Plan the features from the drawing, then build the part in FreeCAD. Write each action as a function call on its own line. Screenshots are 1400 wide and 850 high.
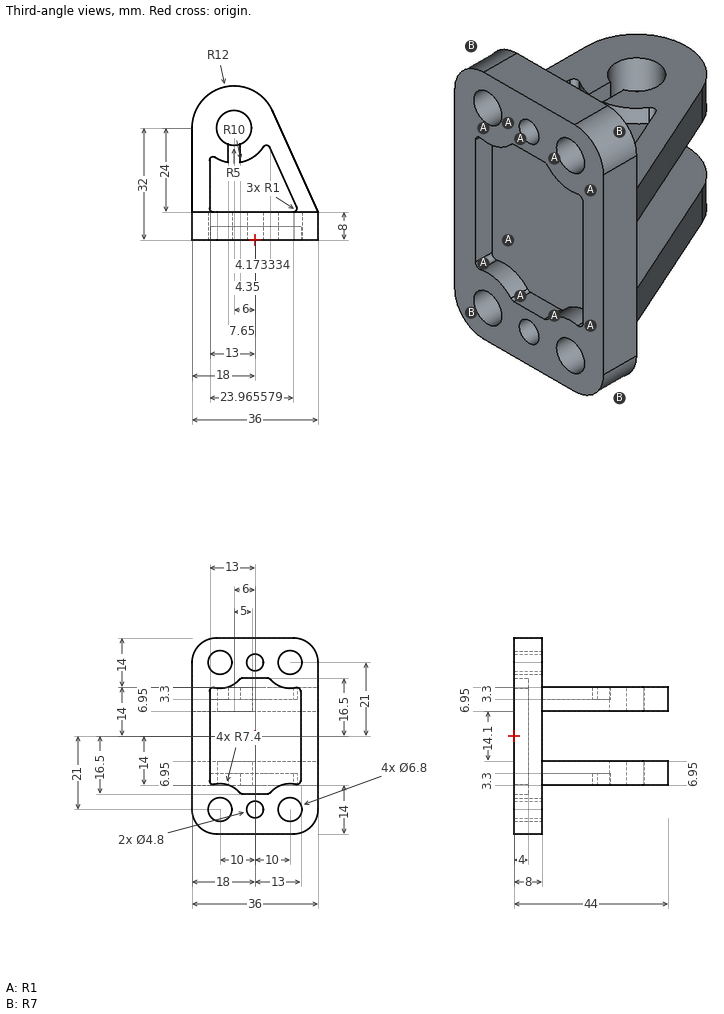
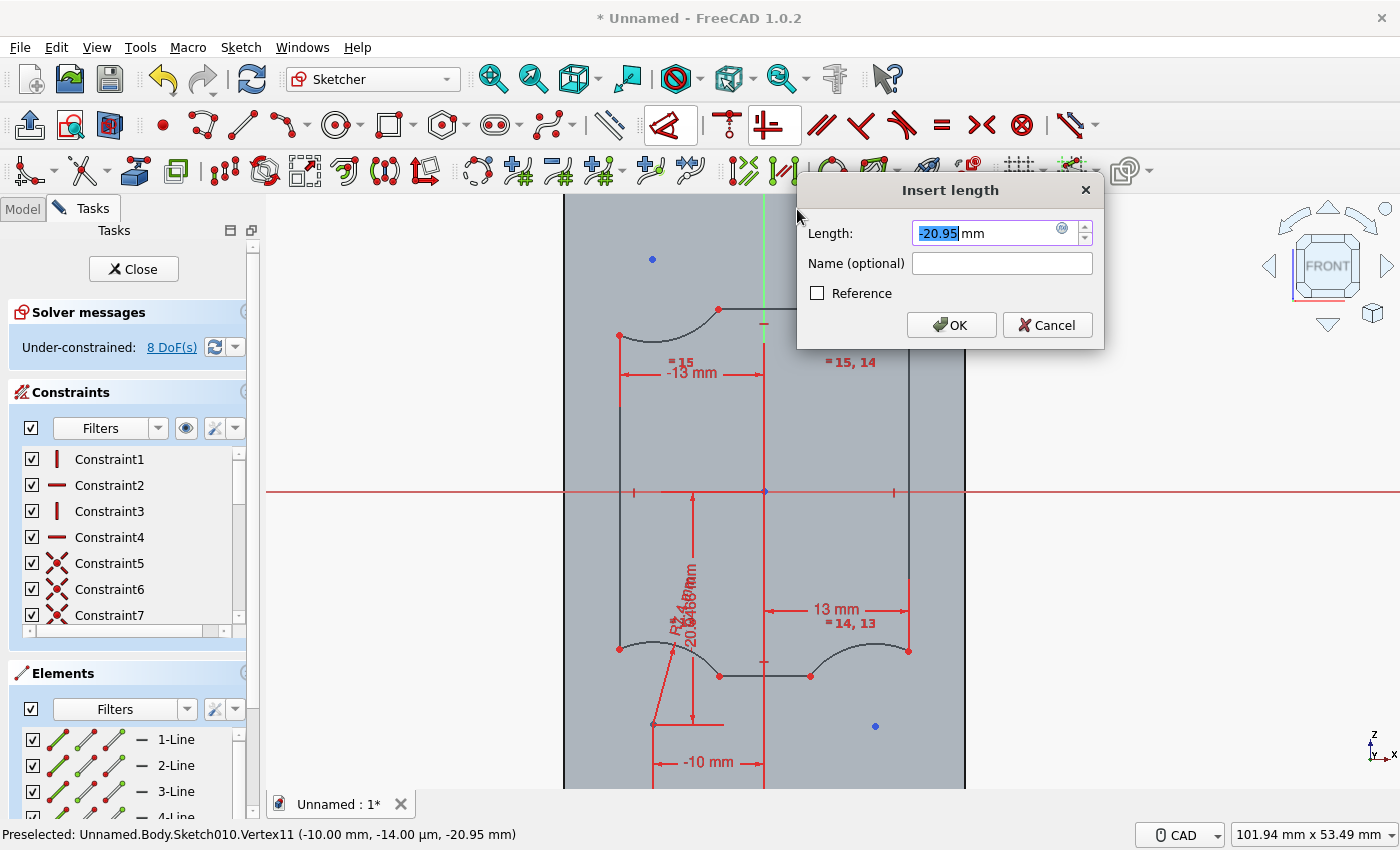
text(-21)
key(Return)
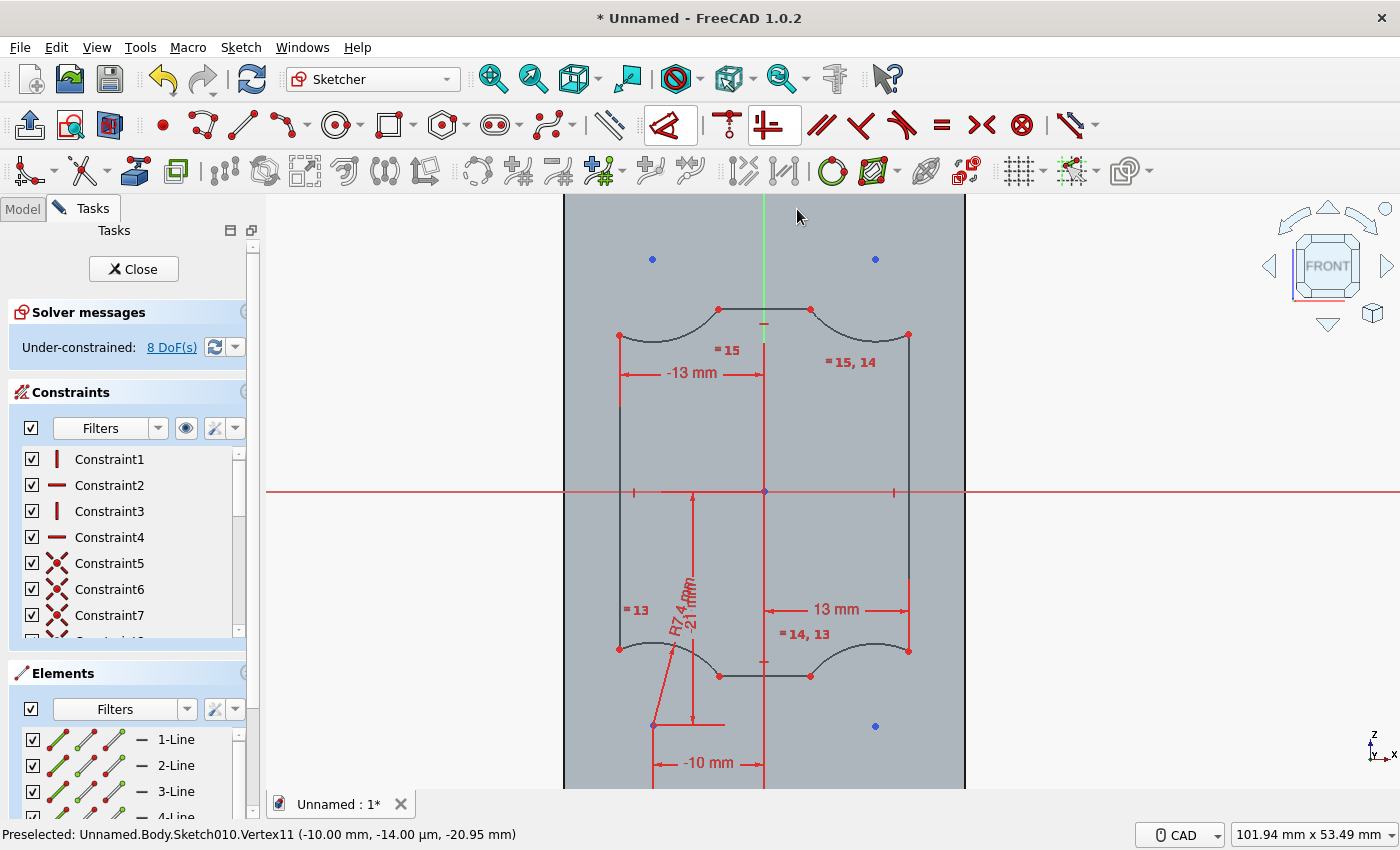
click(875, 726)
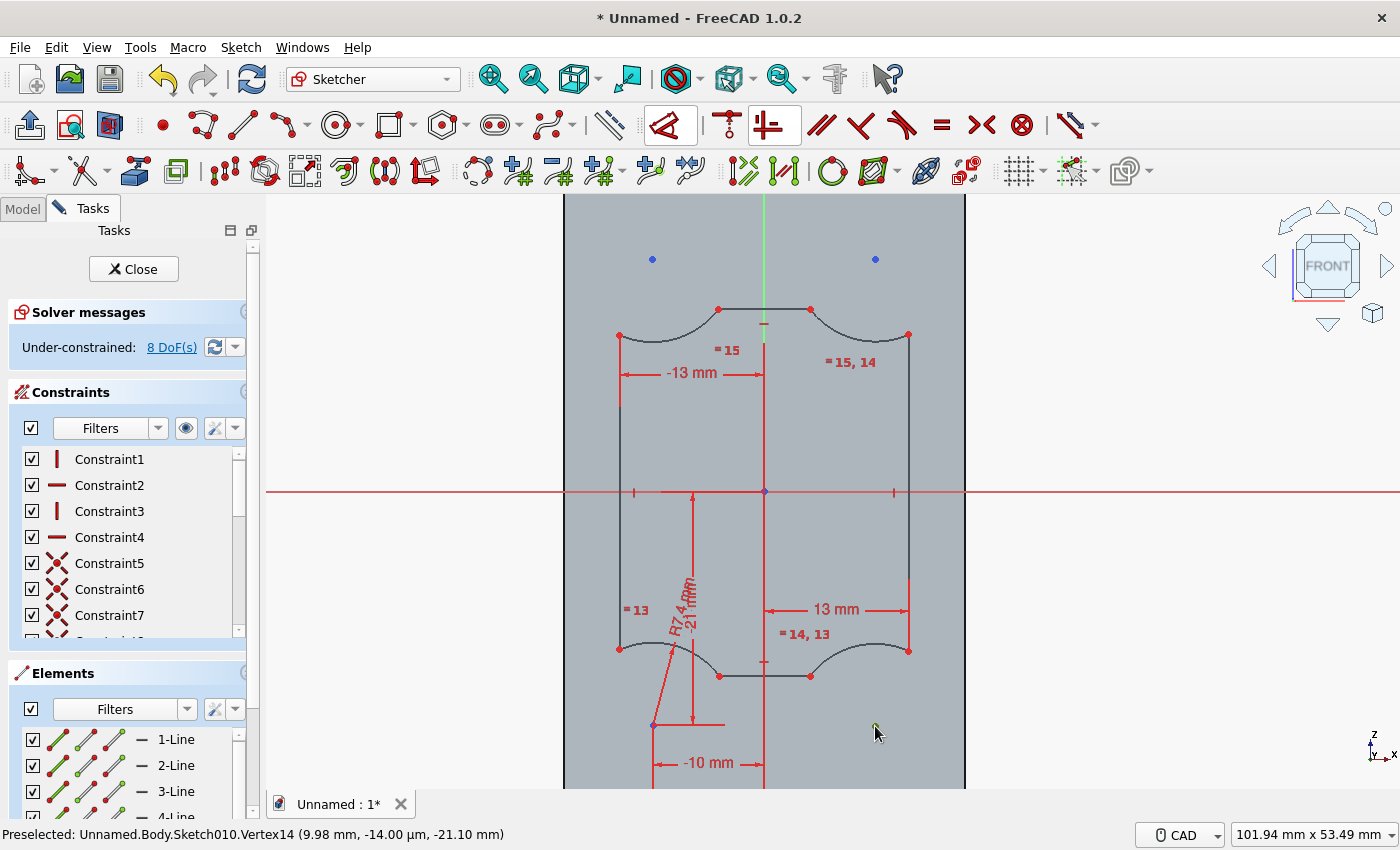
key(l)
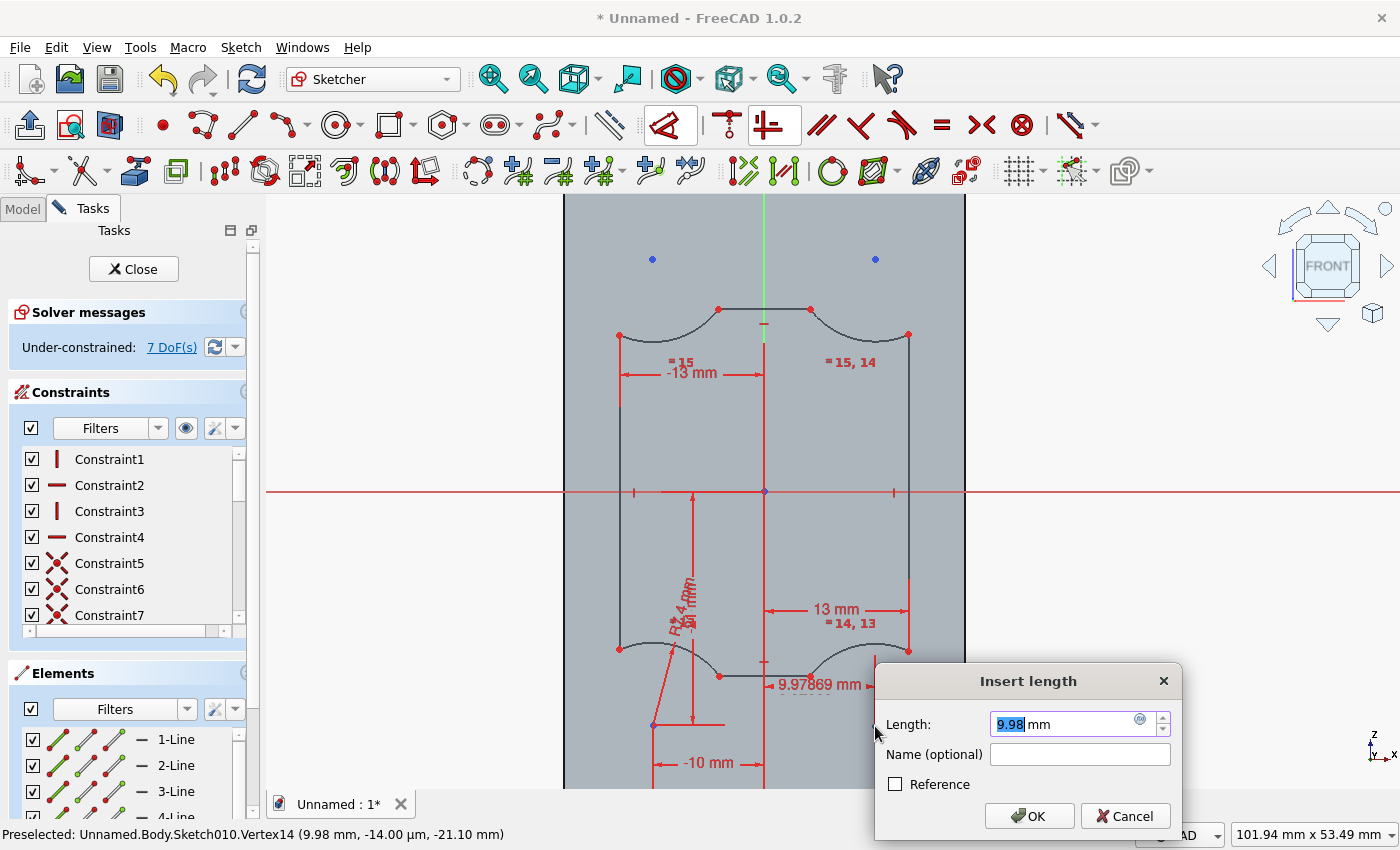
text(10)
key(Return)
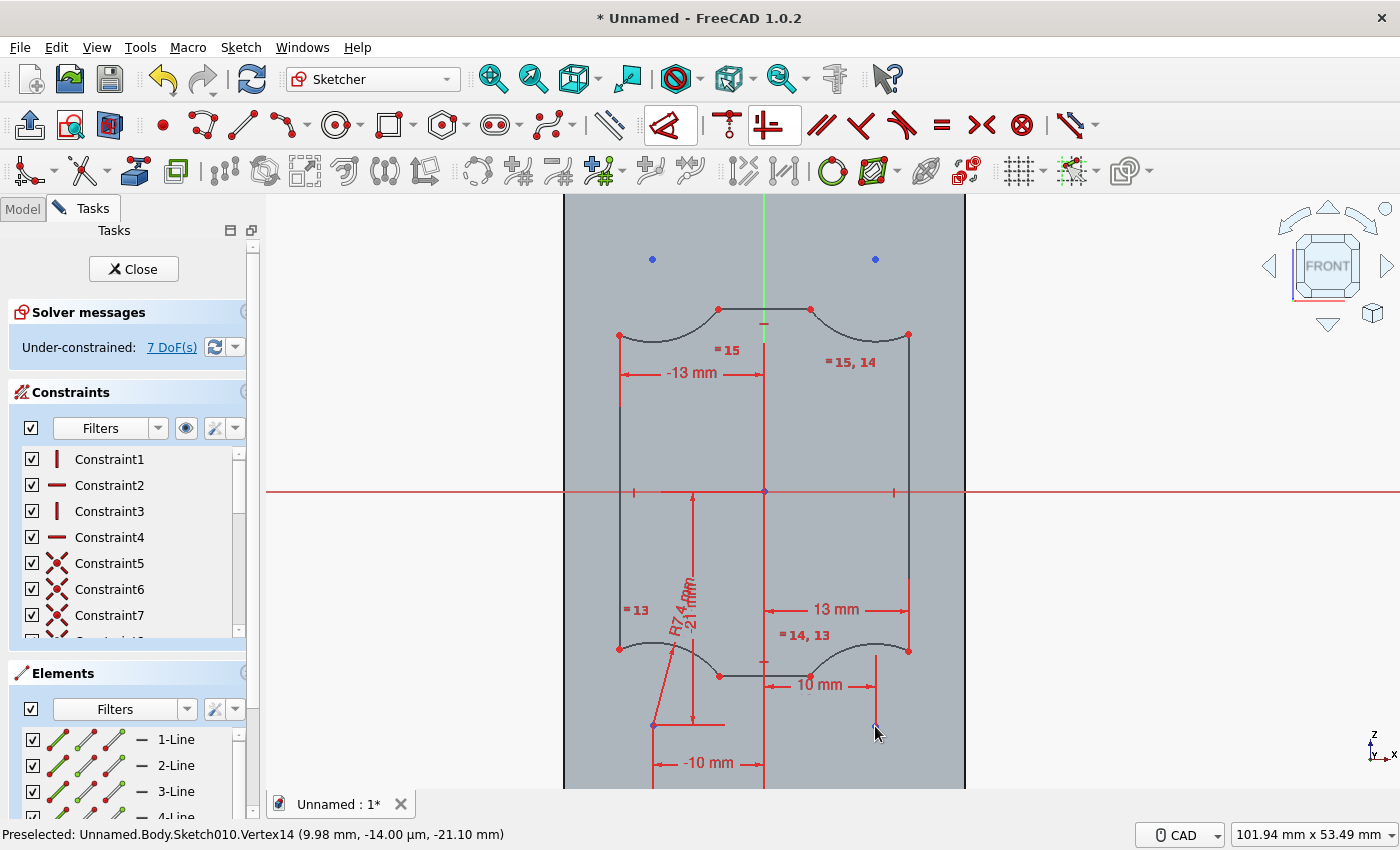
click(876, 726)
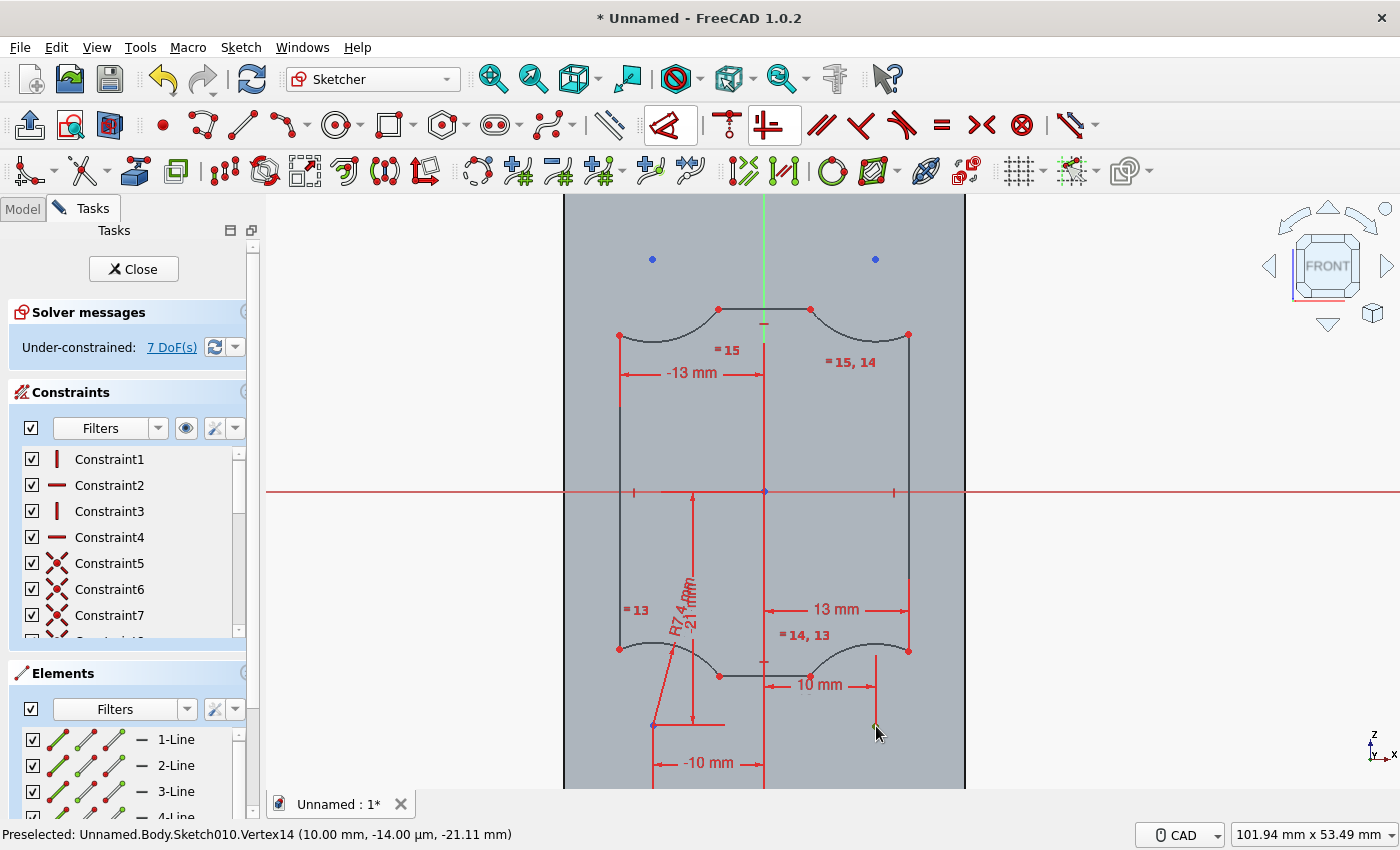
key(i)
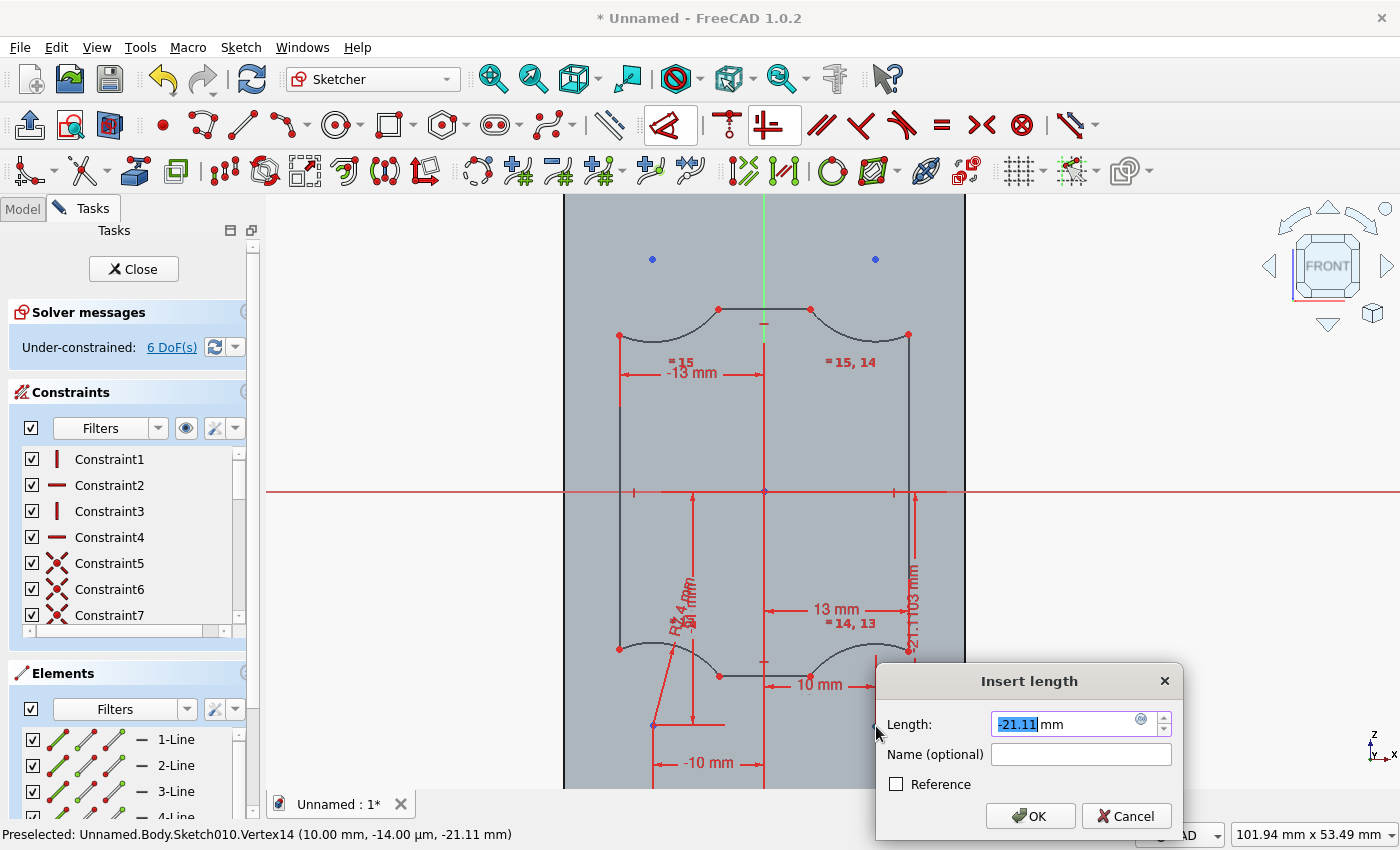
text(-21)
key(Return)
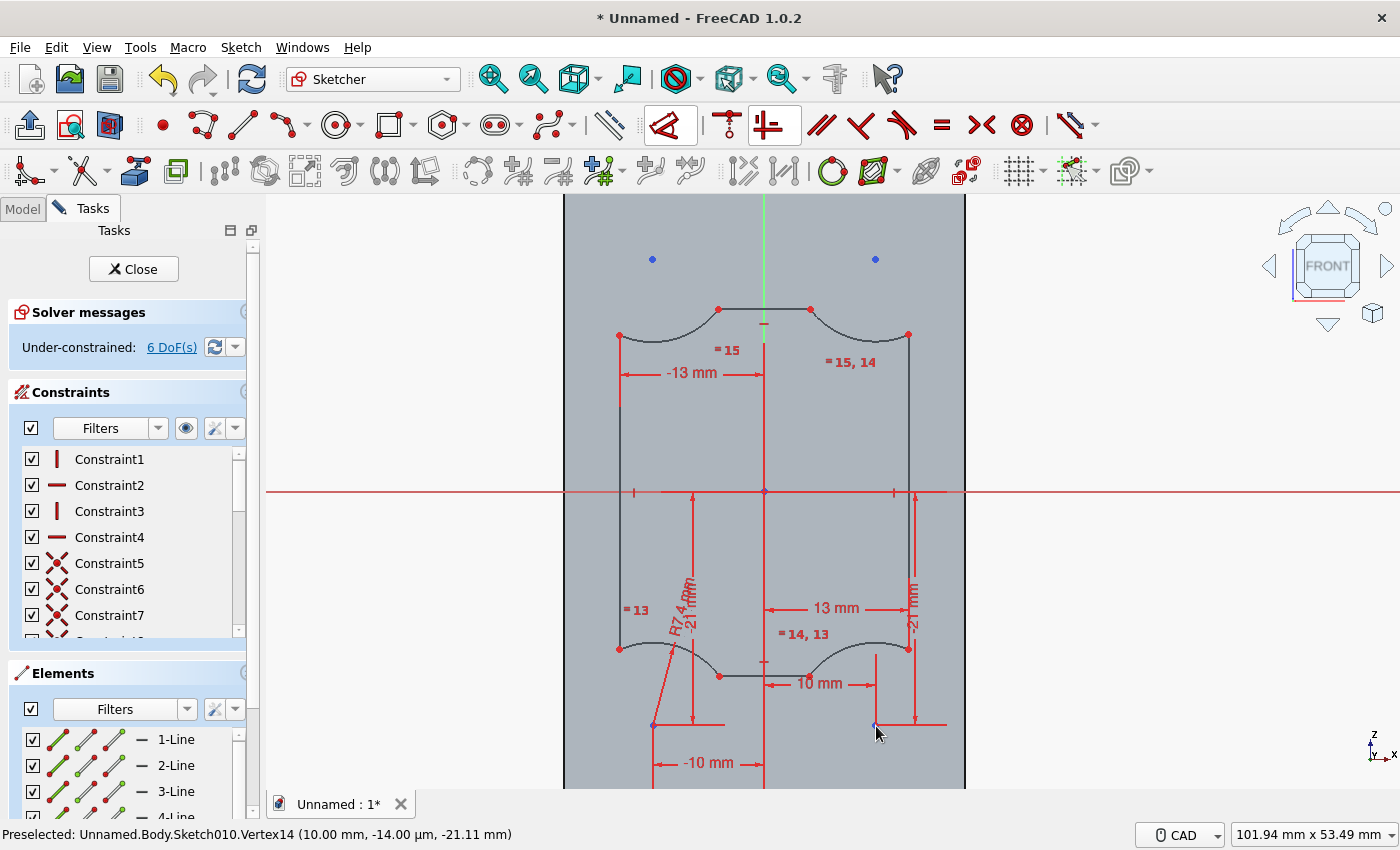
click(876, 259)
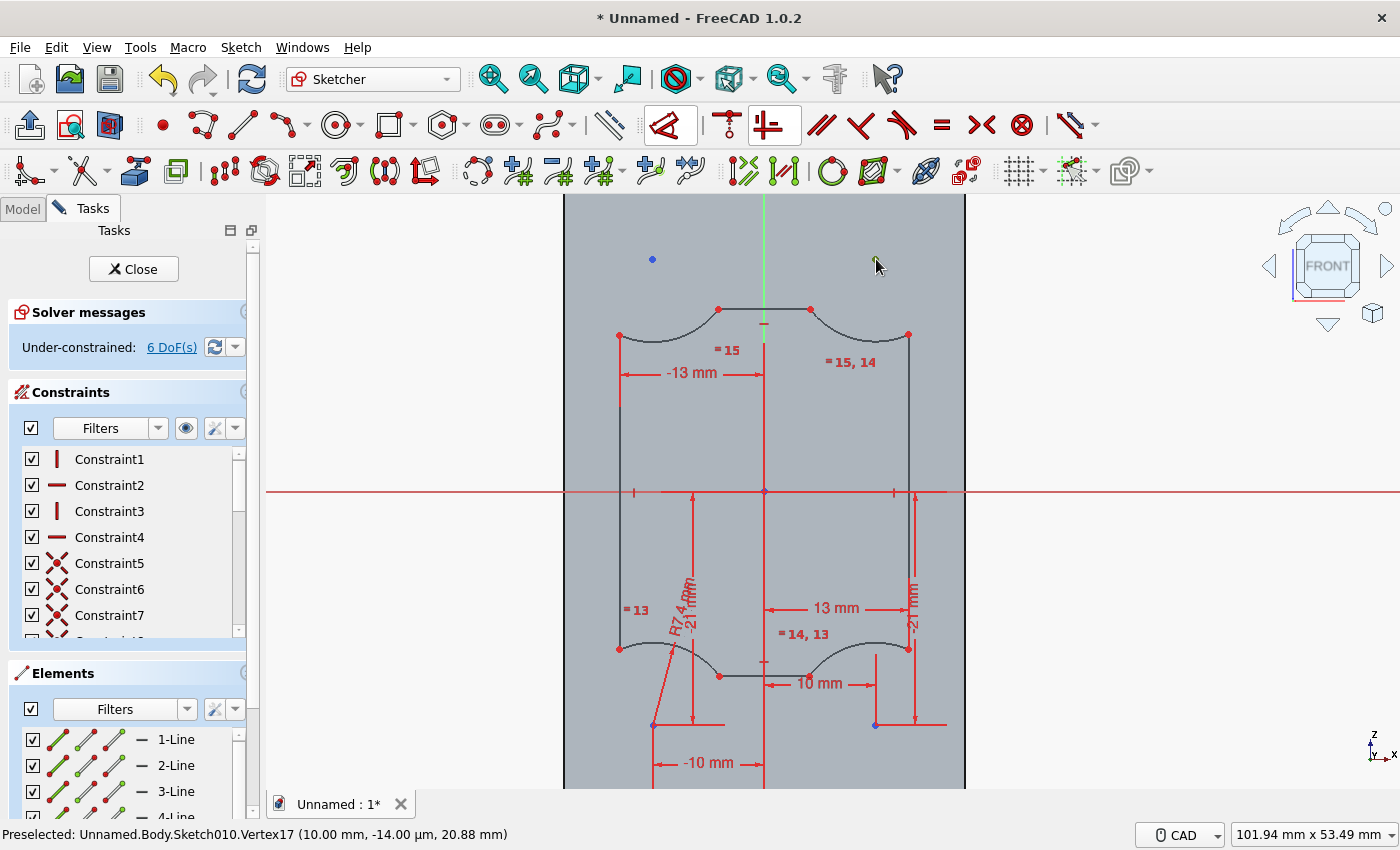
click(692, 126)